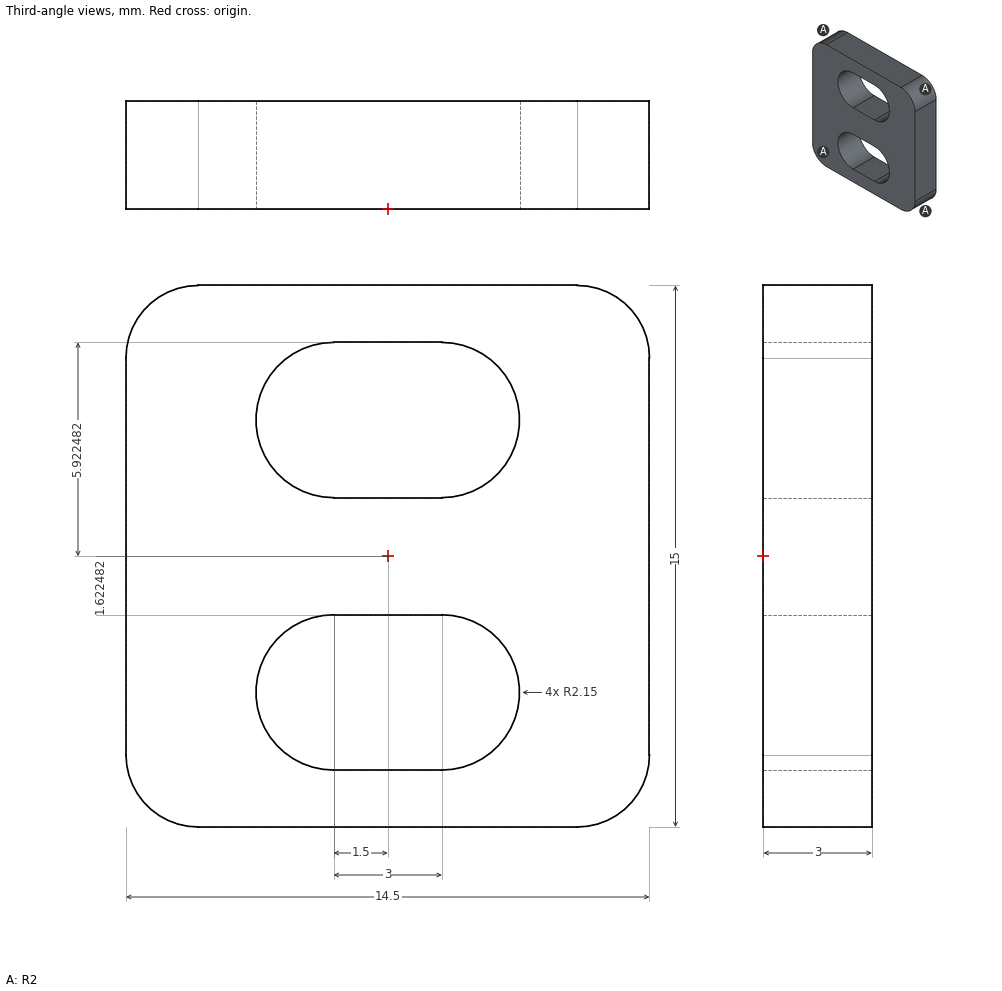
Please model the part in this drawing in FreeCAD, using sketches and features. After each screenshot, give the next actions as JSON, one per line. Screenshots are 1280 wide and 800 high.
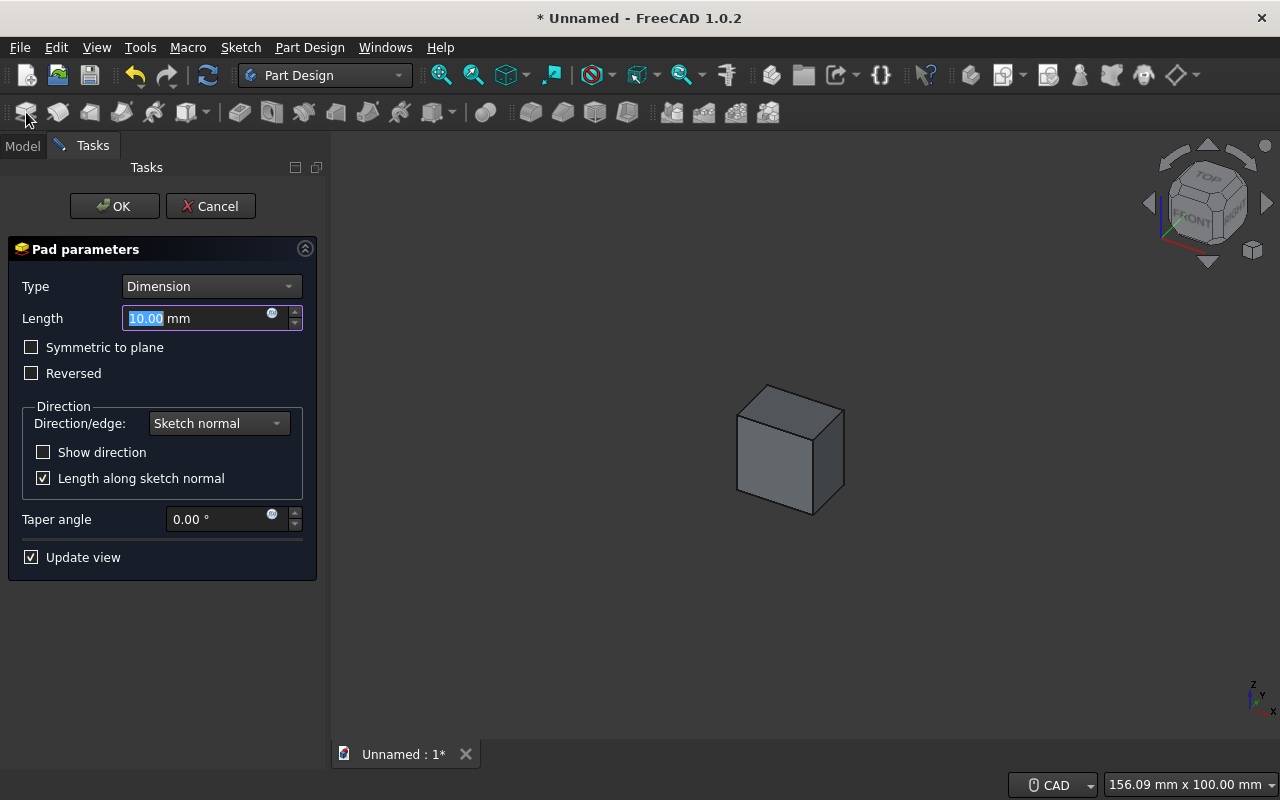
{"action": "type", "text": "3"}
{"action": "key", "text": "Tab"}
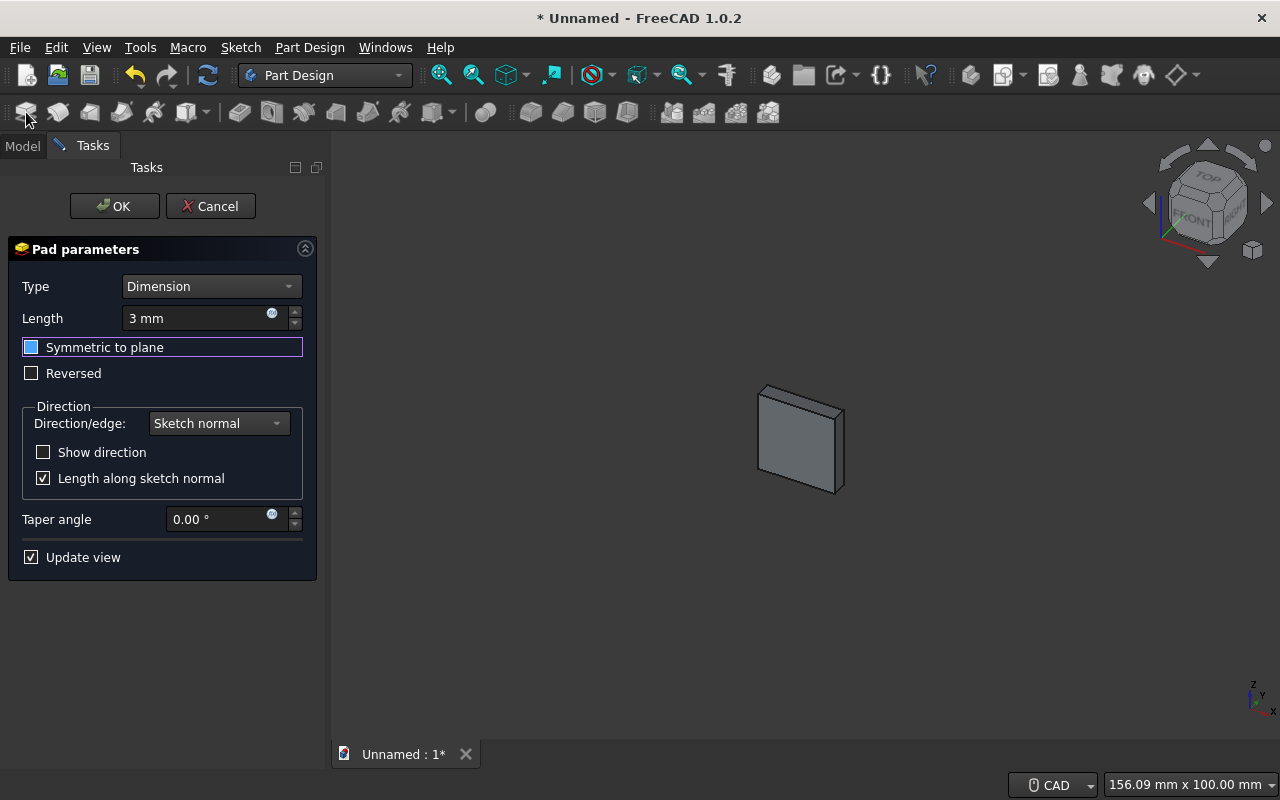
{"action": "left_click", "coordinate": [30, 373]}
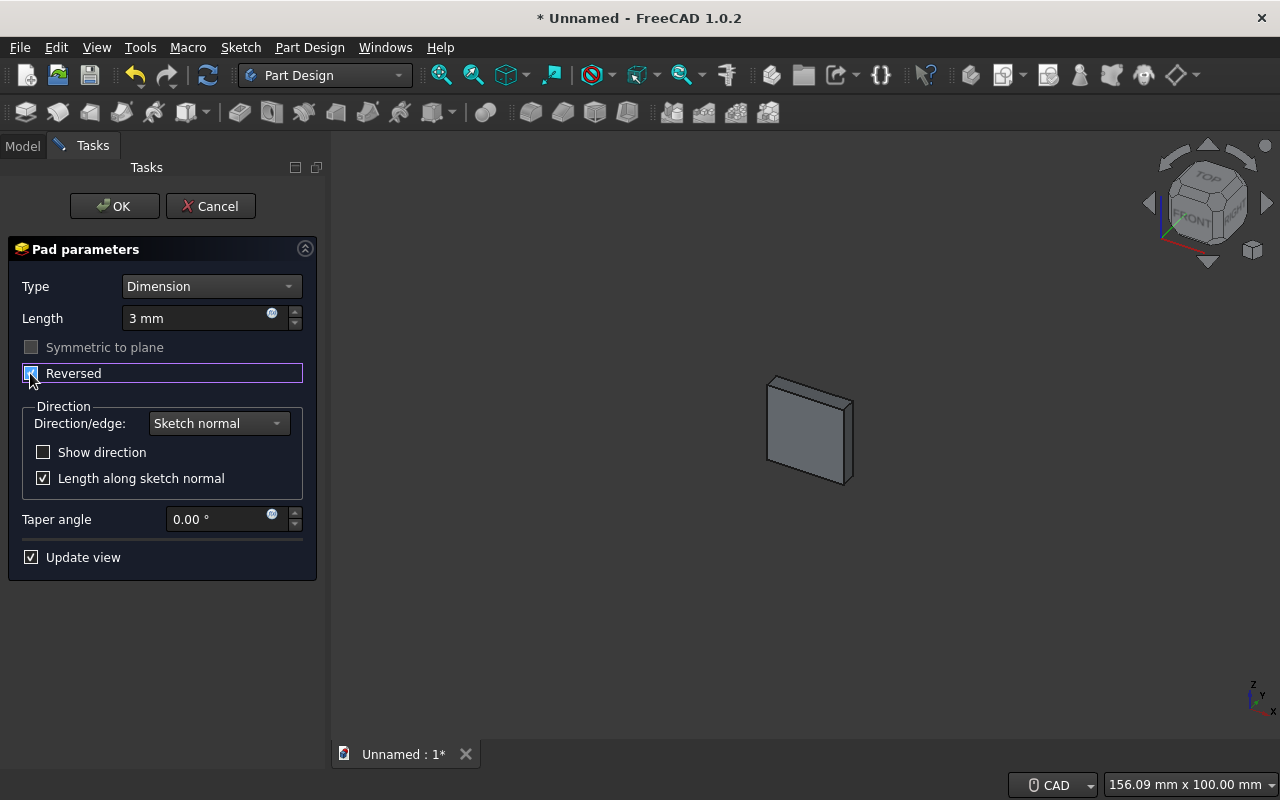
{"action": "left_click", "coordinate": [115, 206]}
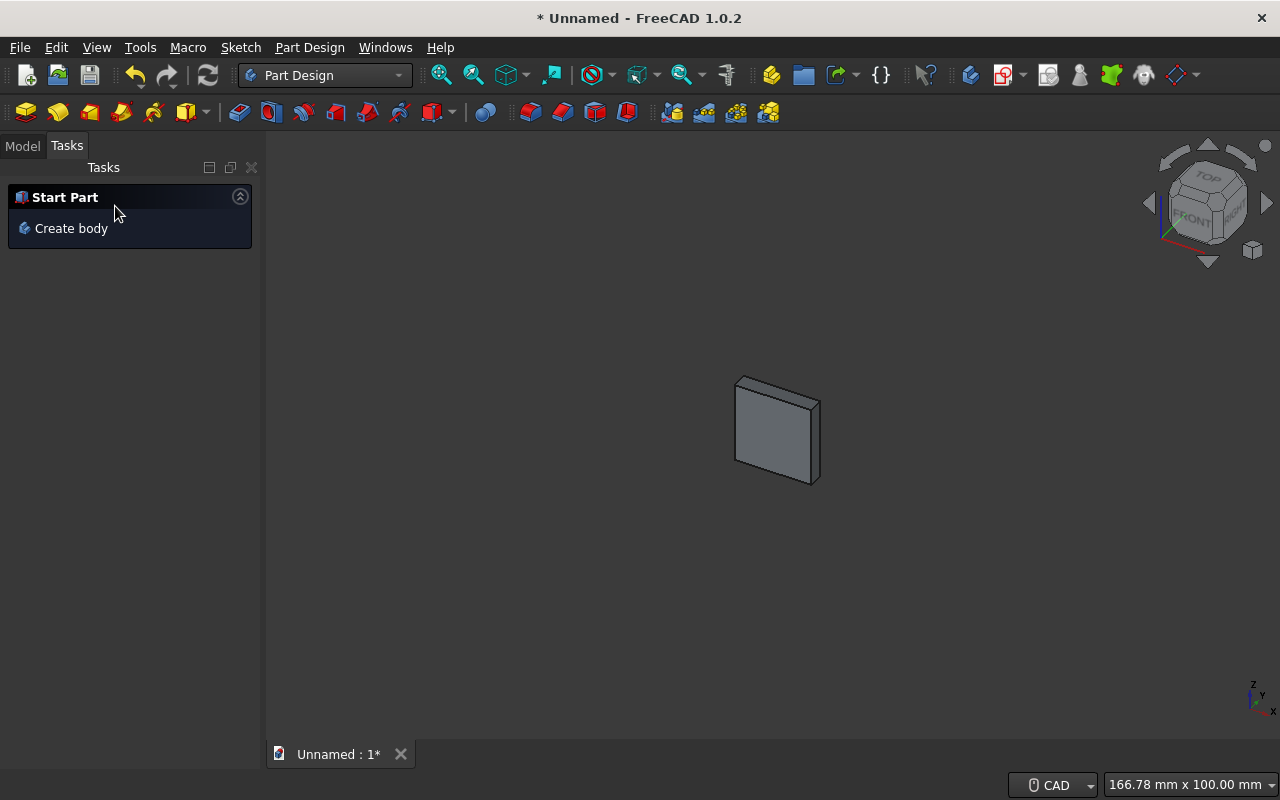
{"action": "left_click", "coordinate": [442, 76]}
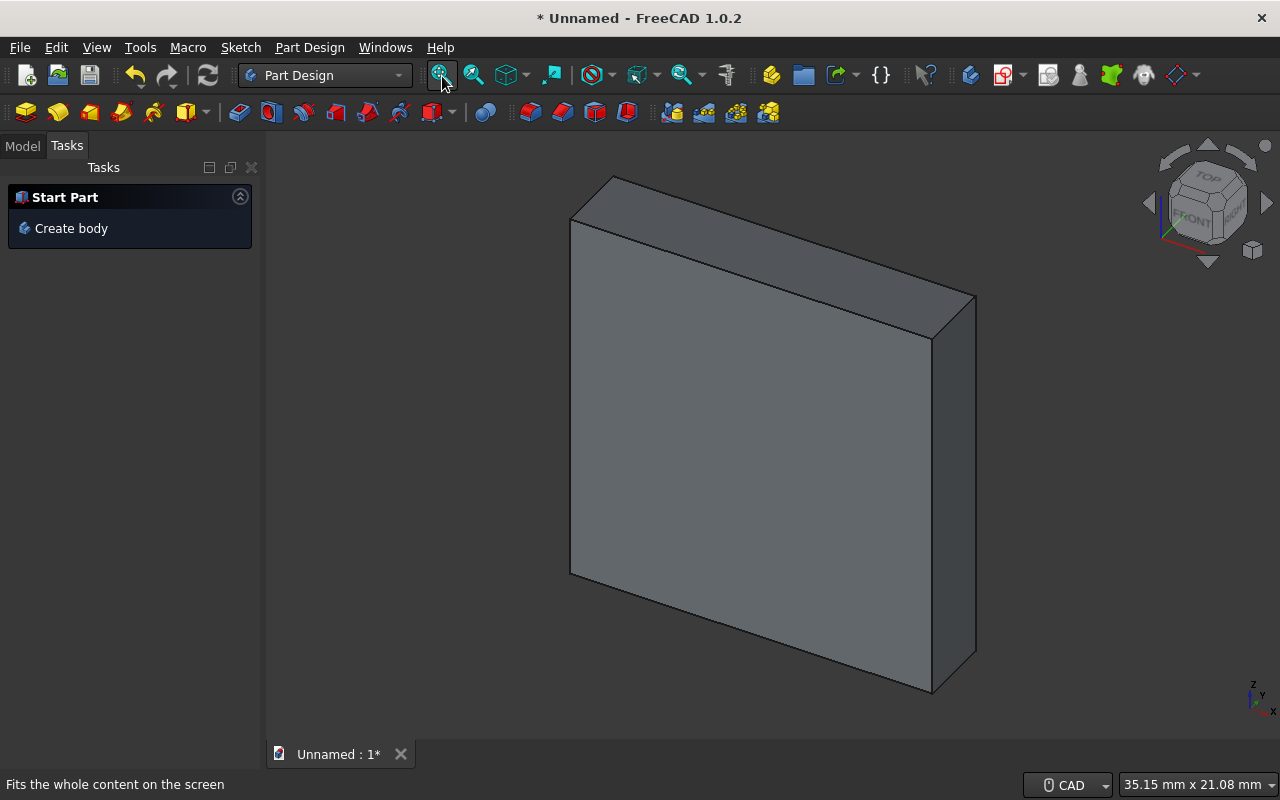
{"action": "left_click", "coordinate": [1004, 76]}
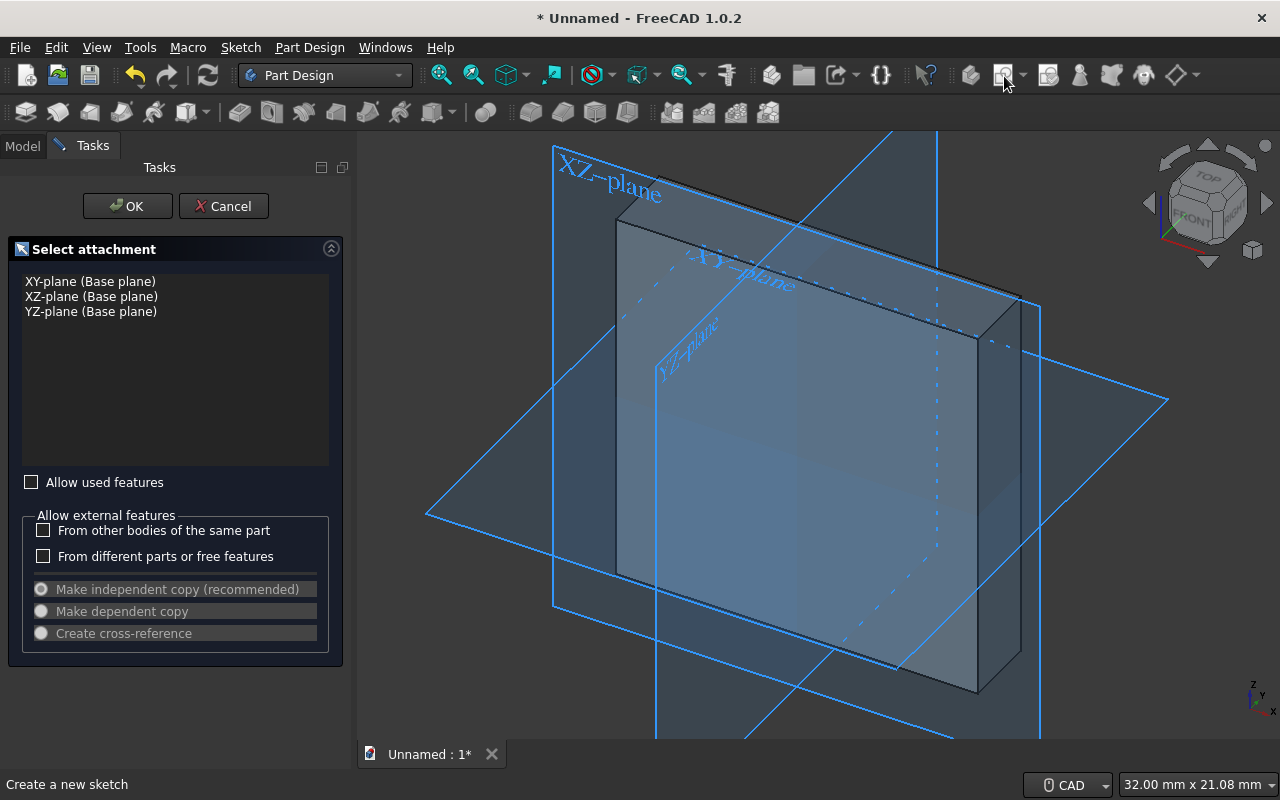
{"action": "left_click", "coordinate": [82, 296]}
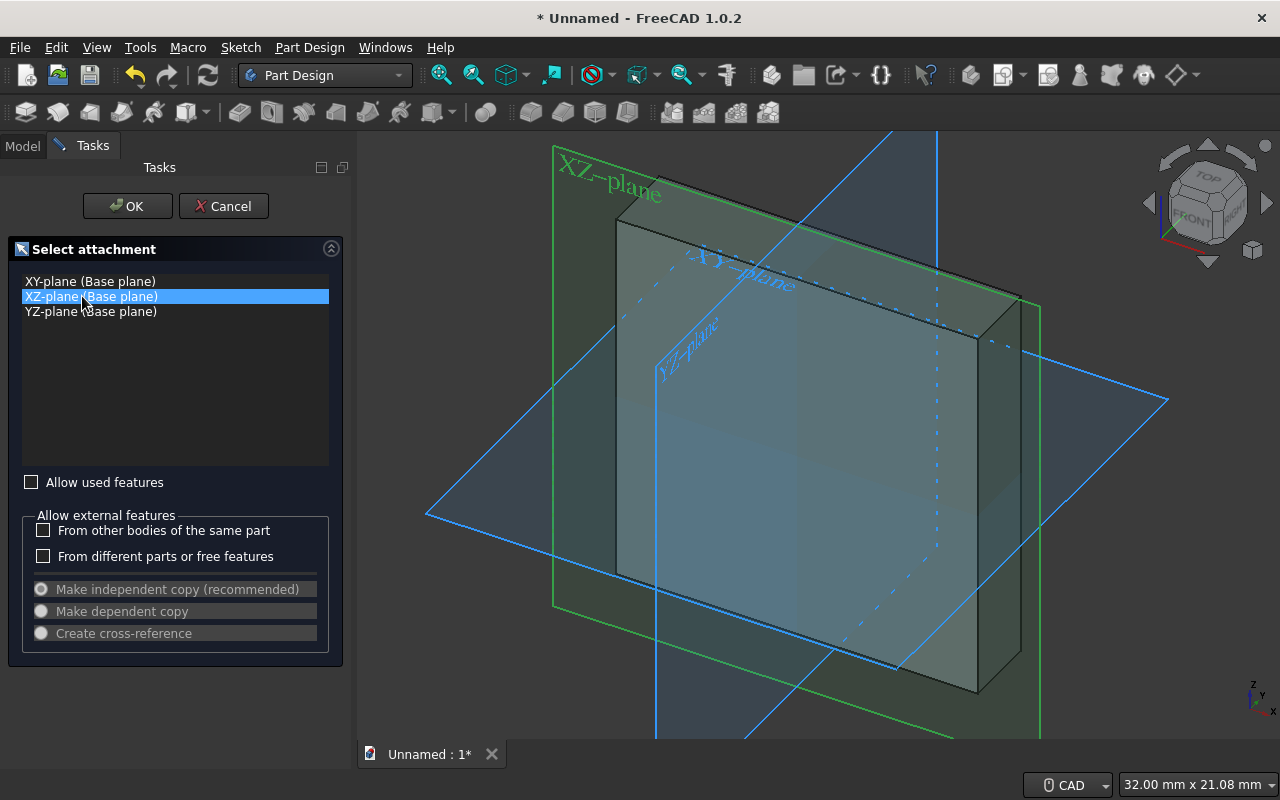
{"action": "left_click", "coordinate": [128, 206]}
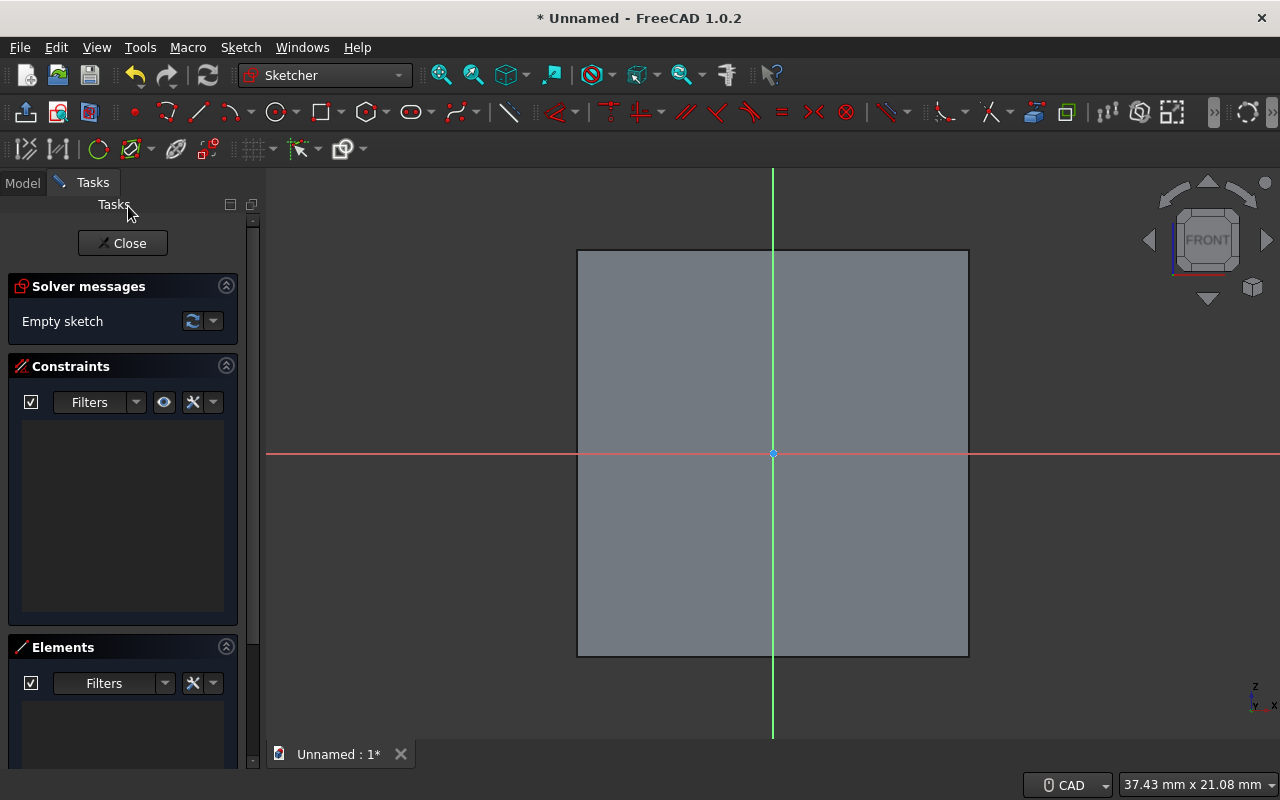
{"action": "left_click", "coordinate": [412, 112]}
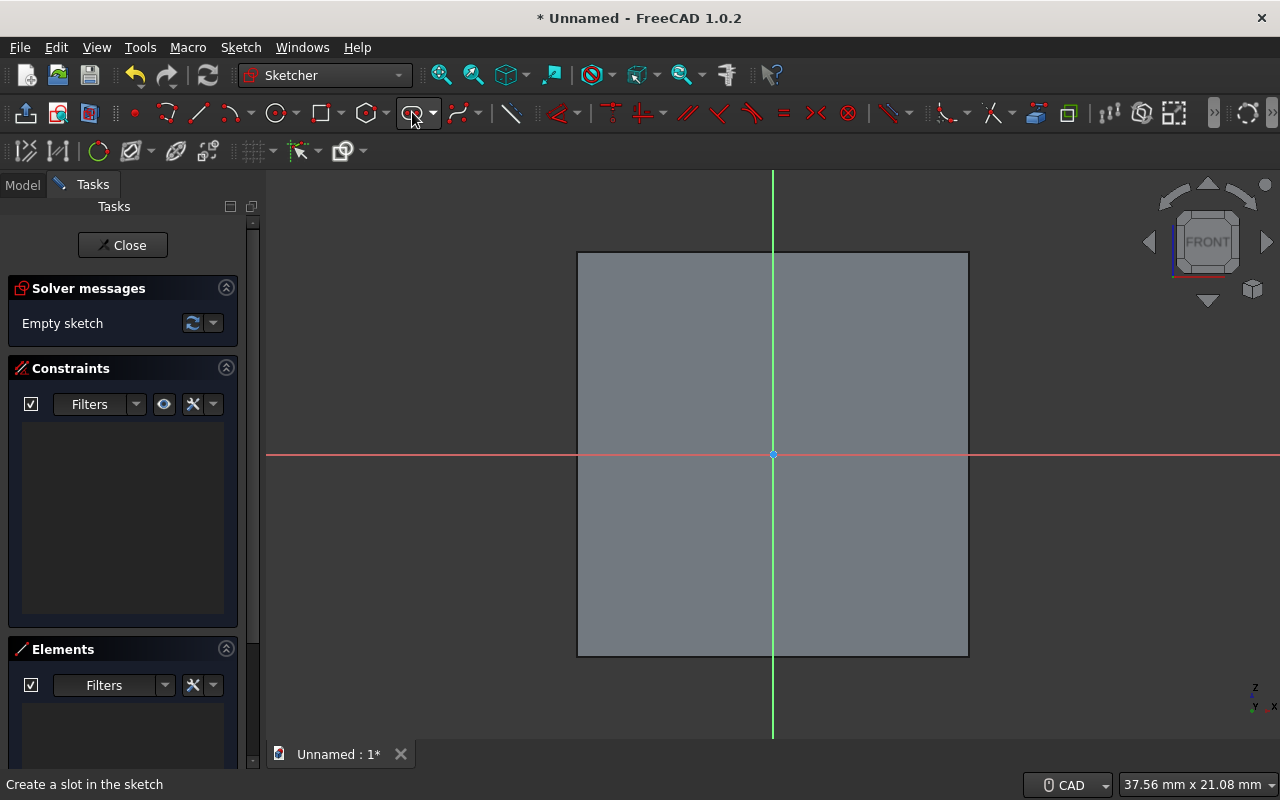
{"action": "left_click", "coordinate": [733, 556]}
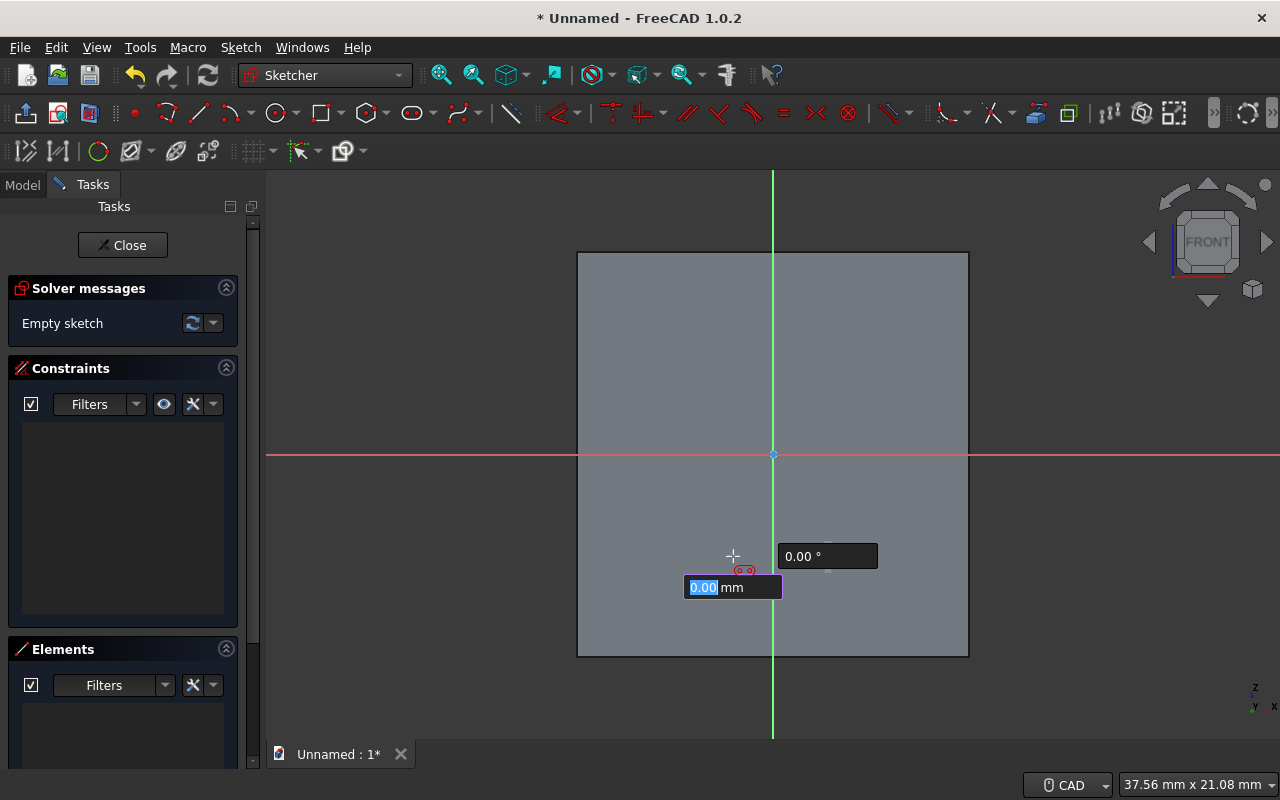
{"action": "left_click", "coordinate": [813, 556]}